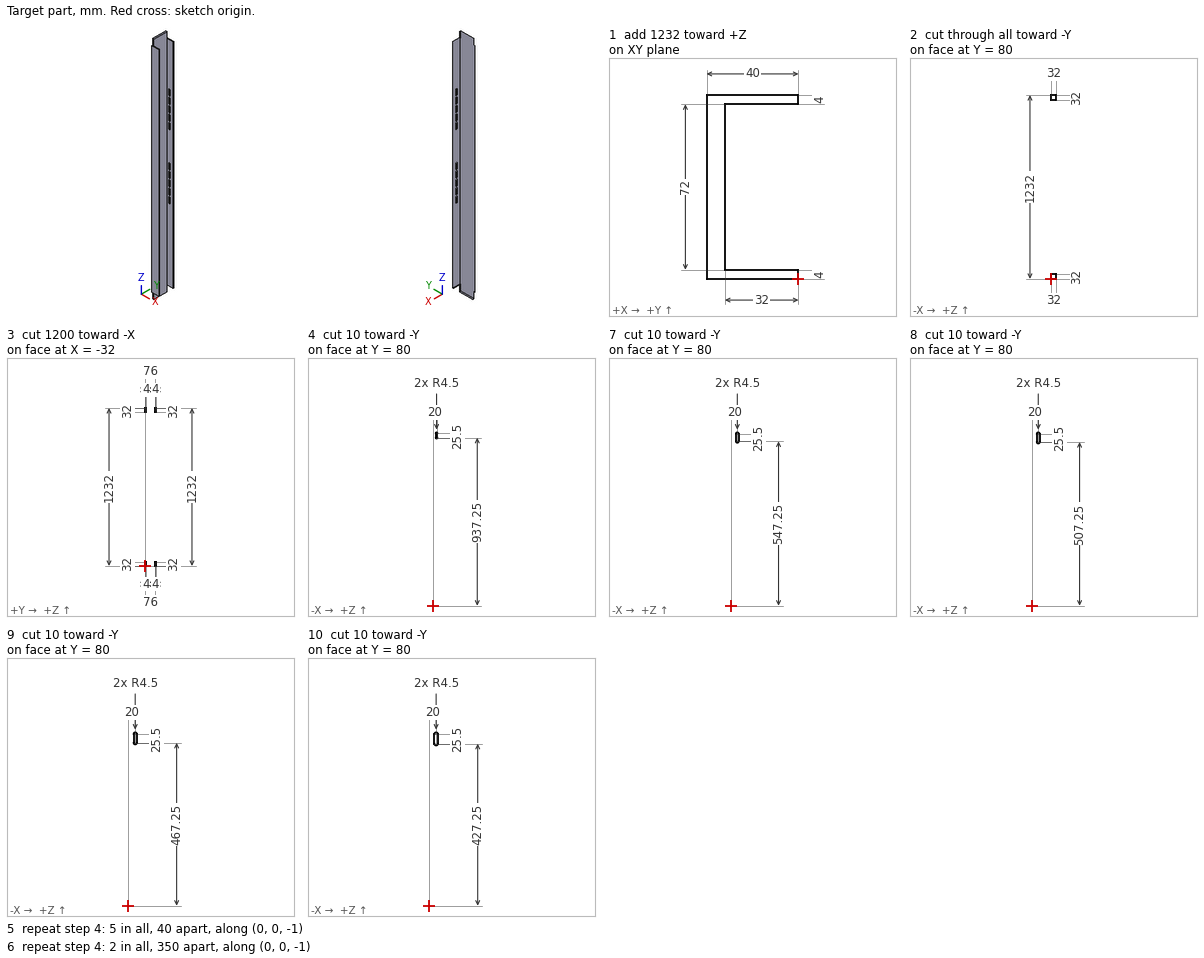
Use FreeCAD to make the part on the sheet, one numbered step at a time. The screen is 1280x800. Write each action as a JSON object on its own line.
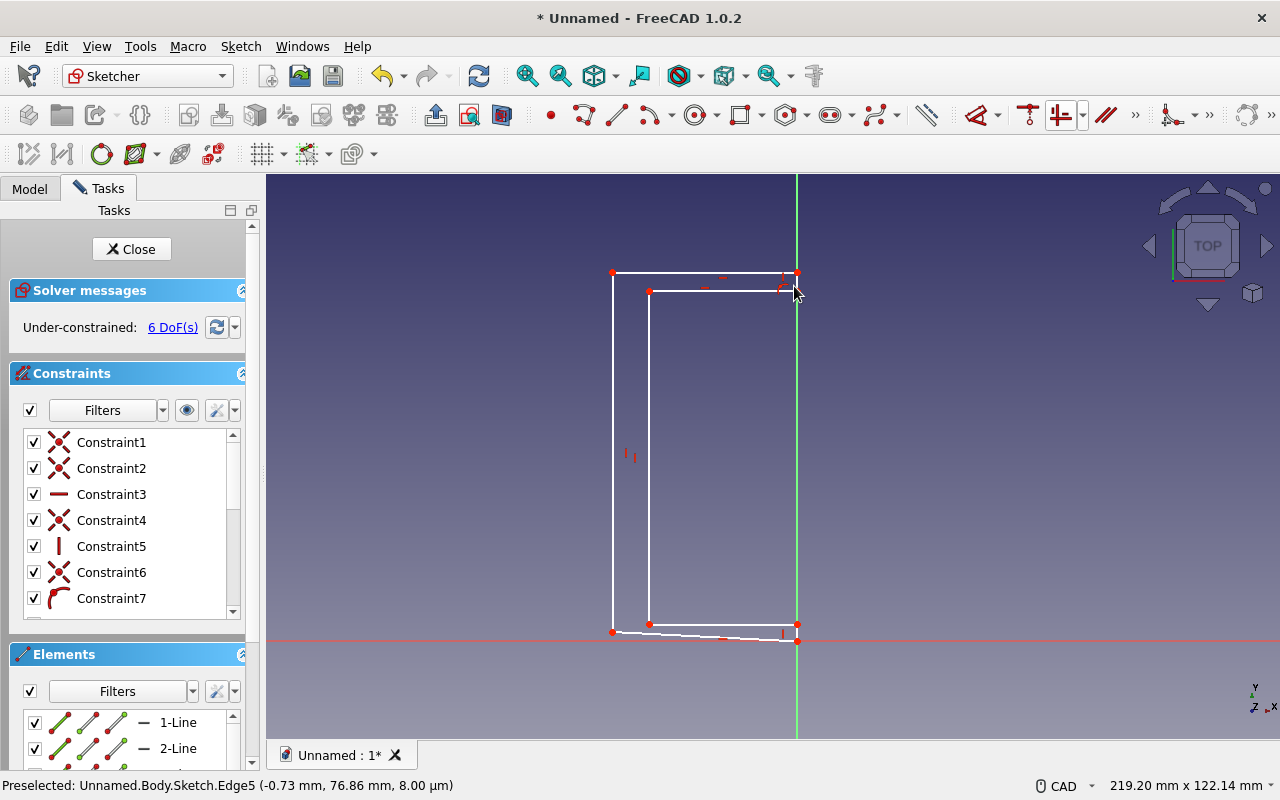
{"action": "scroll", "coordinate": [668, 635], "scroll_direction": "up", "scroll_amount": 4}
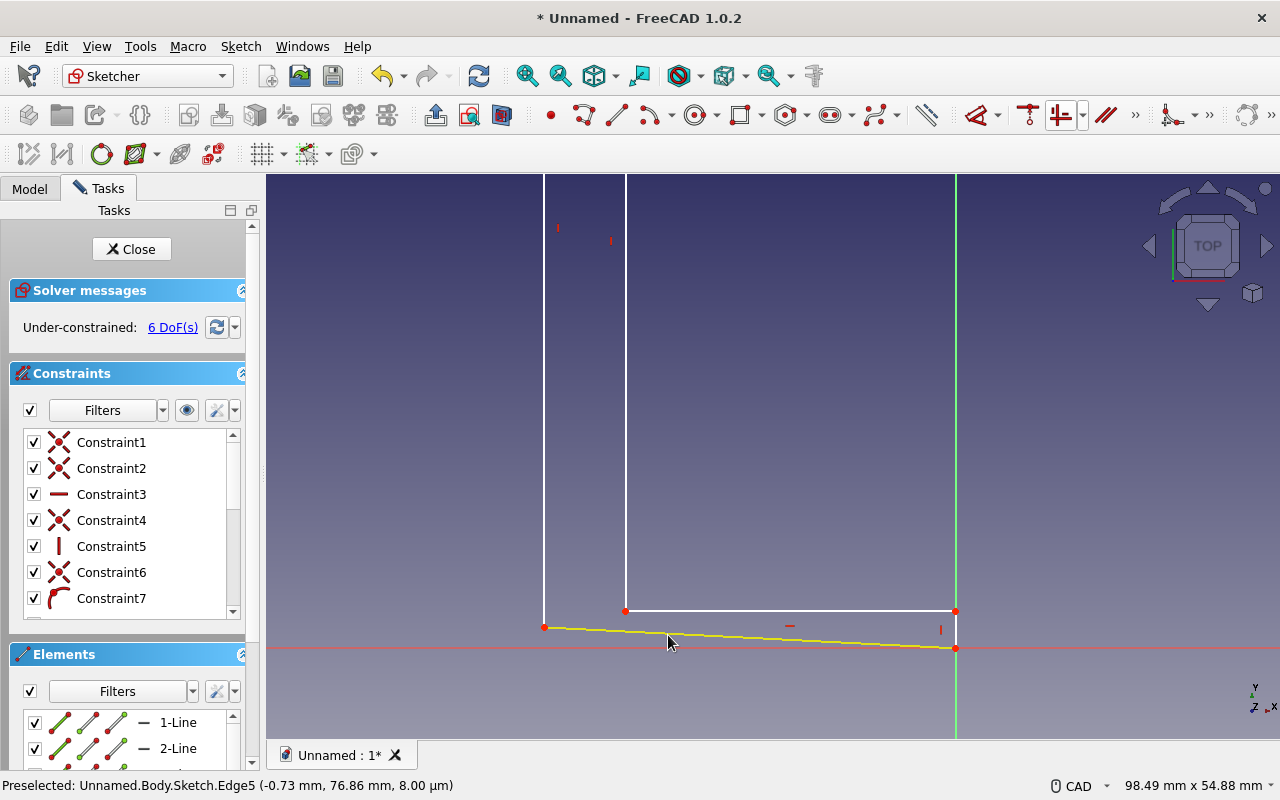
{"action": "left_click", "coordinate": [668, 634]}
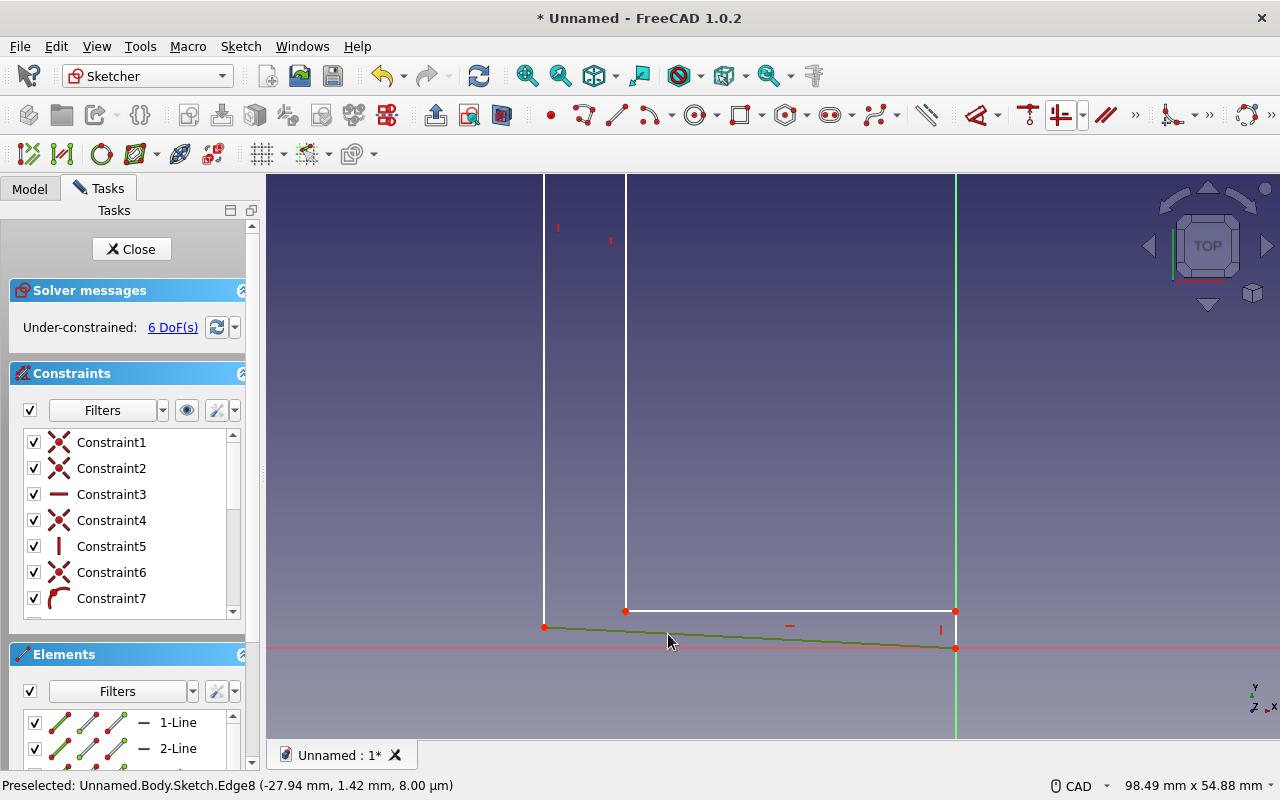
{"action": "left_click", "coordinate": [1082, 116]}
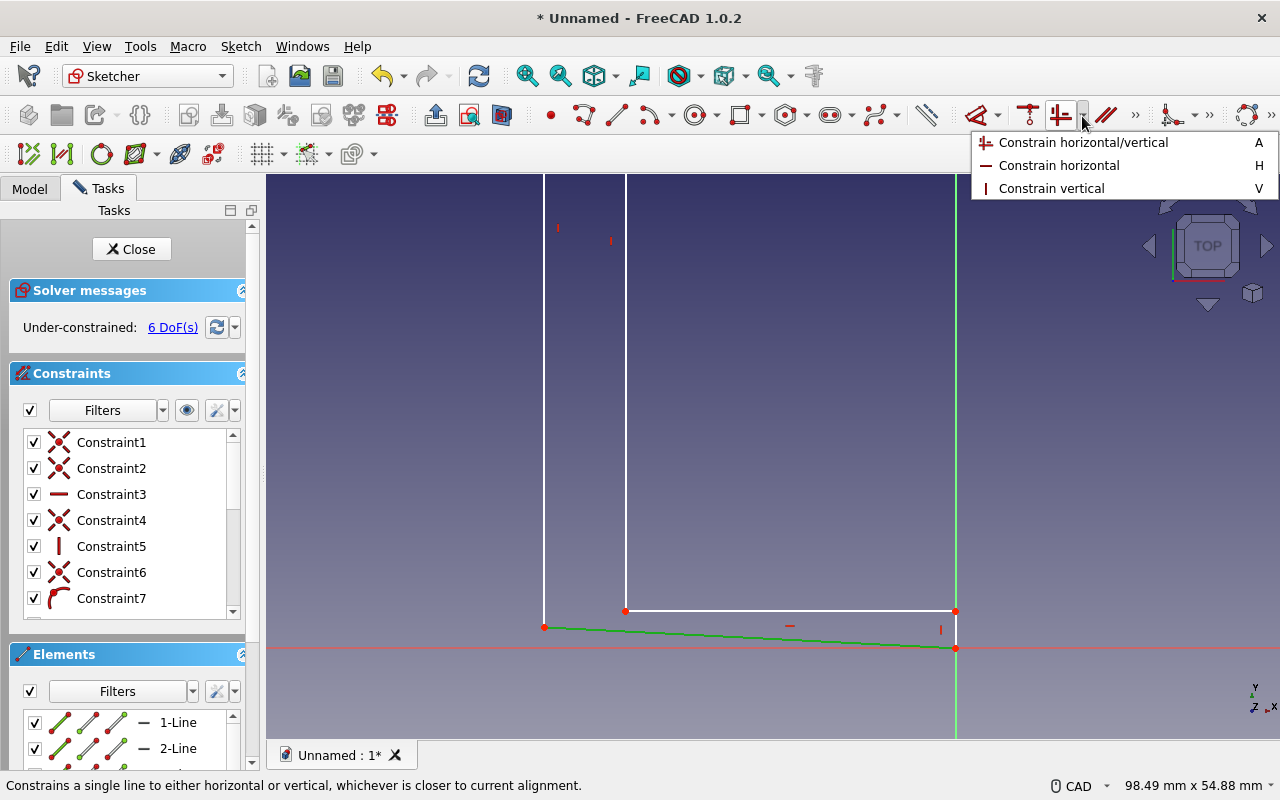
{"action": "left_click", "coordinate": [1125, 166]}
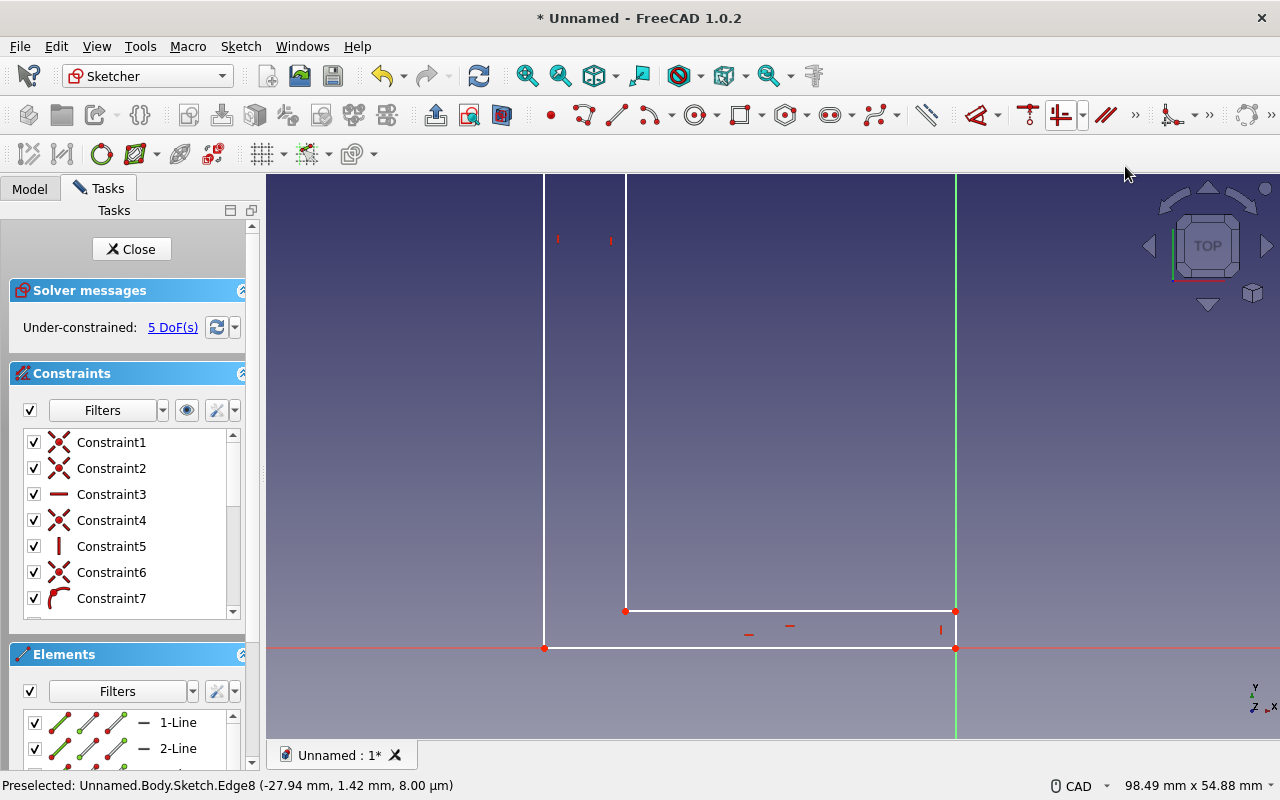
{"action": "scroll", "coordinate": [956, 637], "scroll_direction": "up", "scroll_amount": 2}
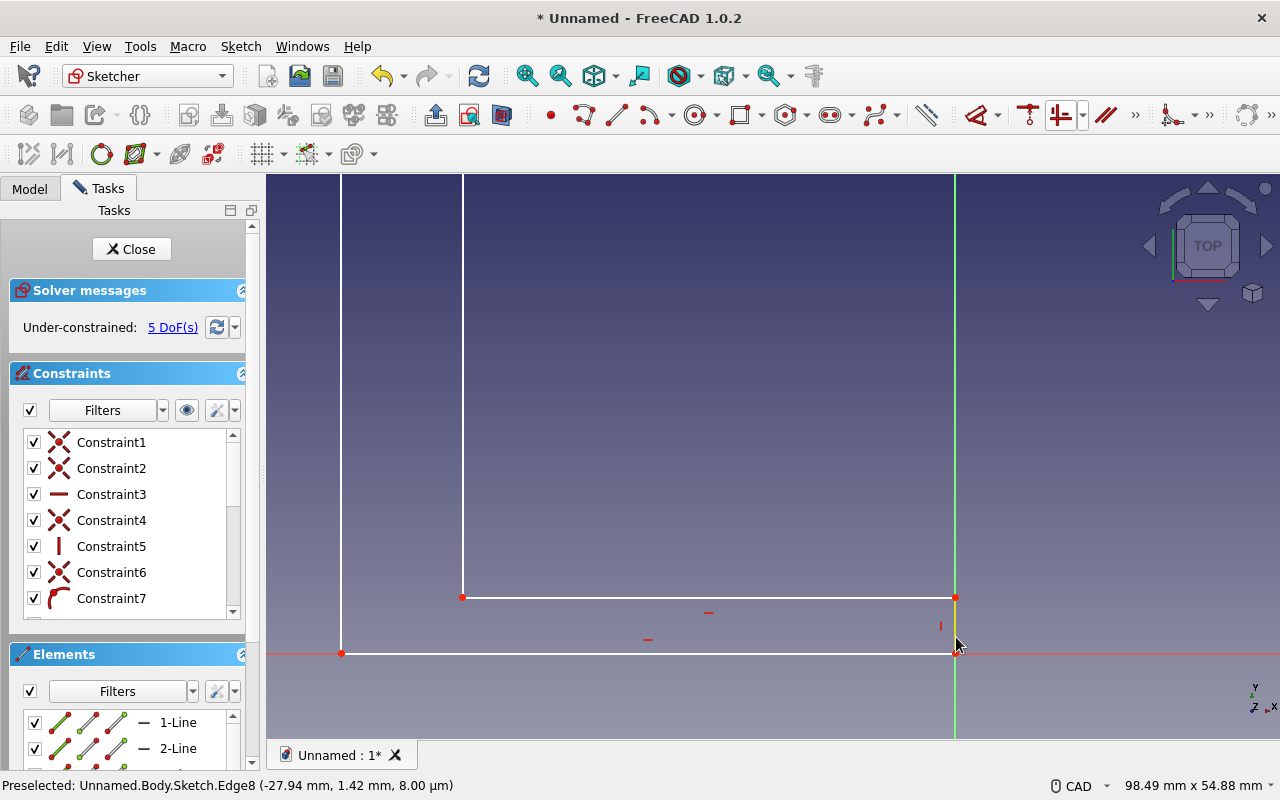
{"action": "left_click", "coordinate": [955, 637]}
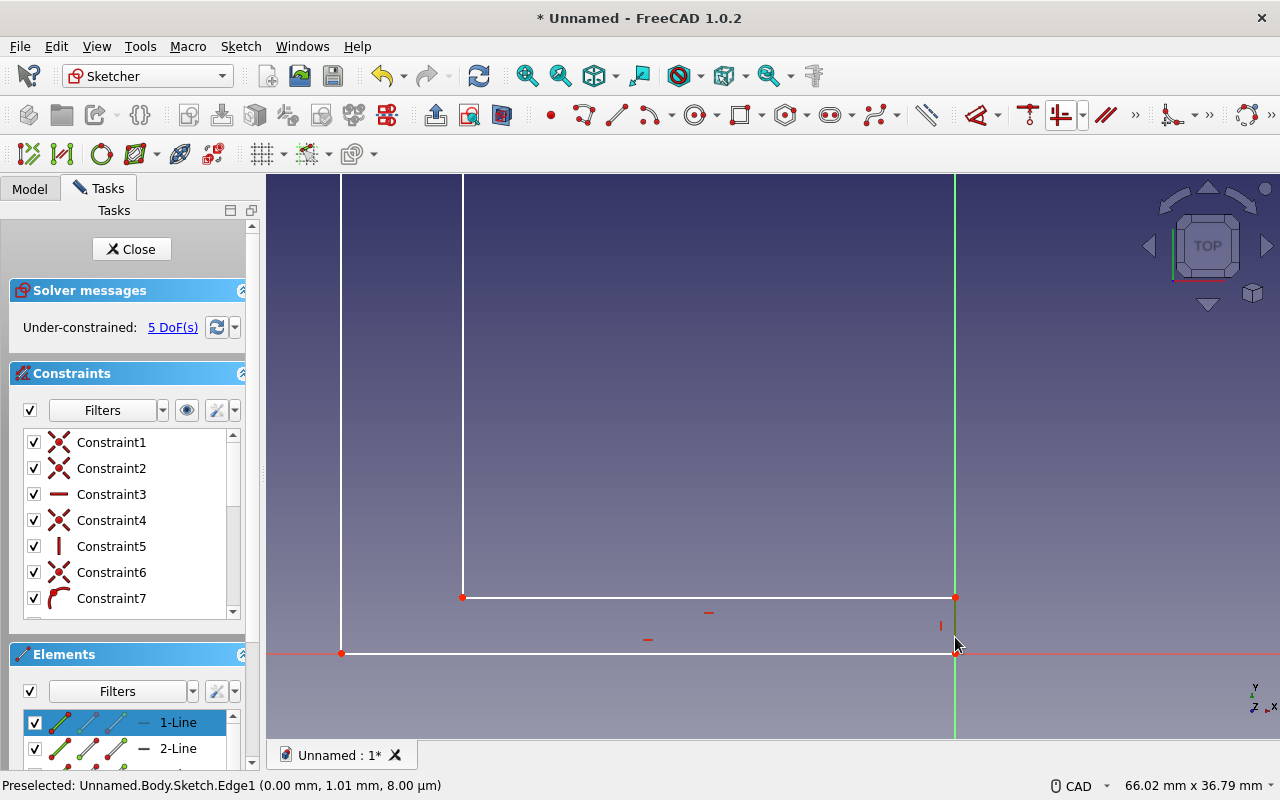
{"action": "left_click", "coordinate": [998, 116]}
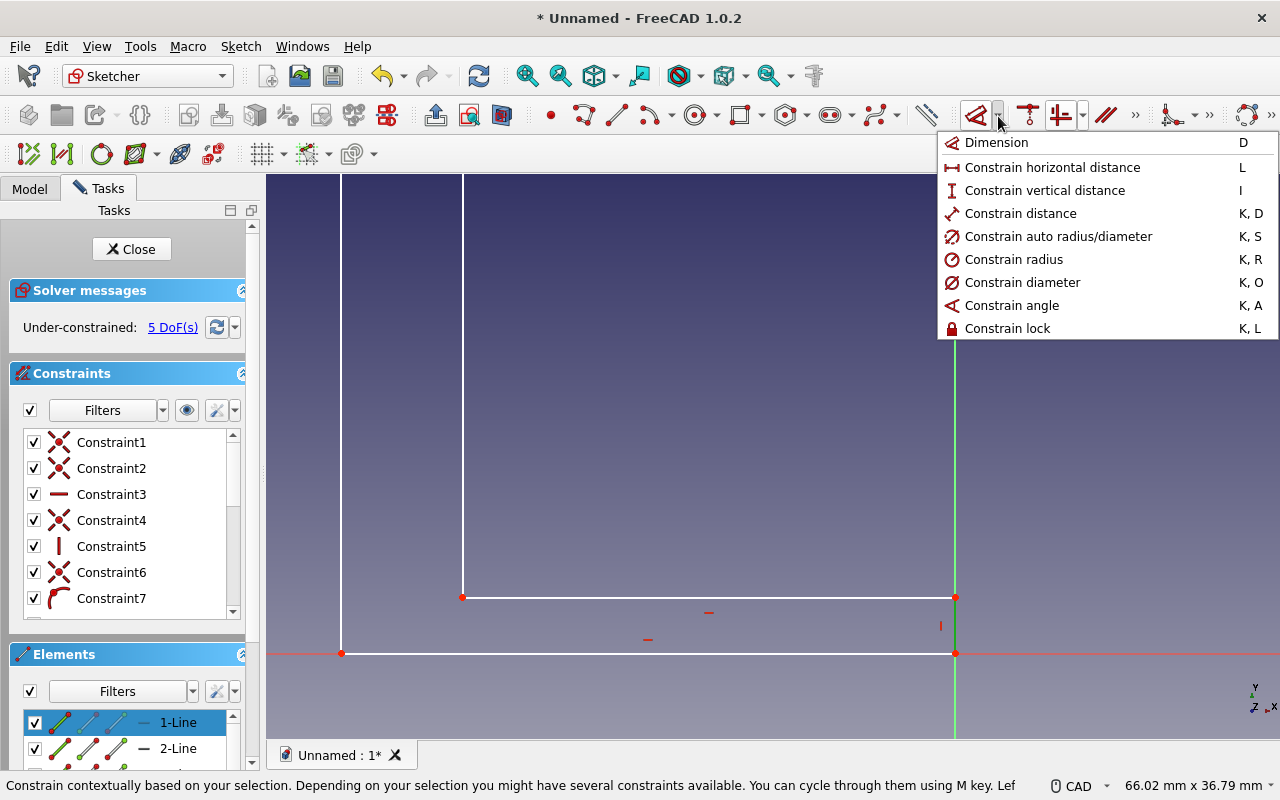
{"action": "left_click", "coordinate": [1108, 190]}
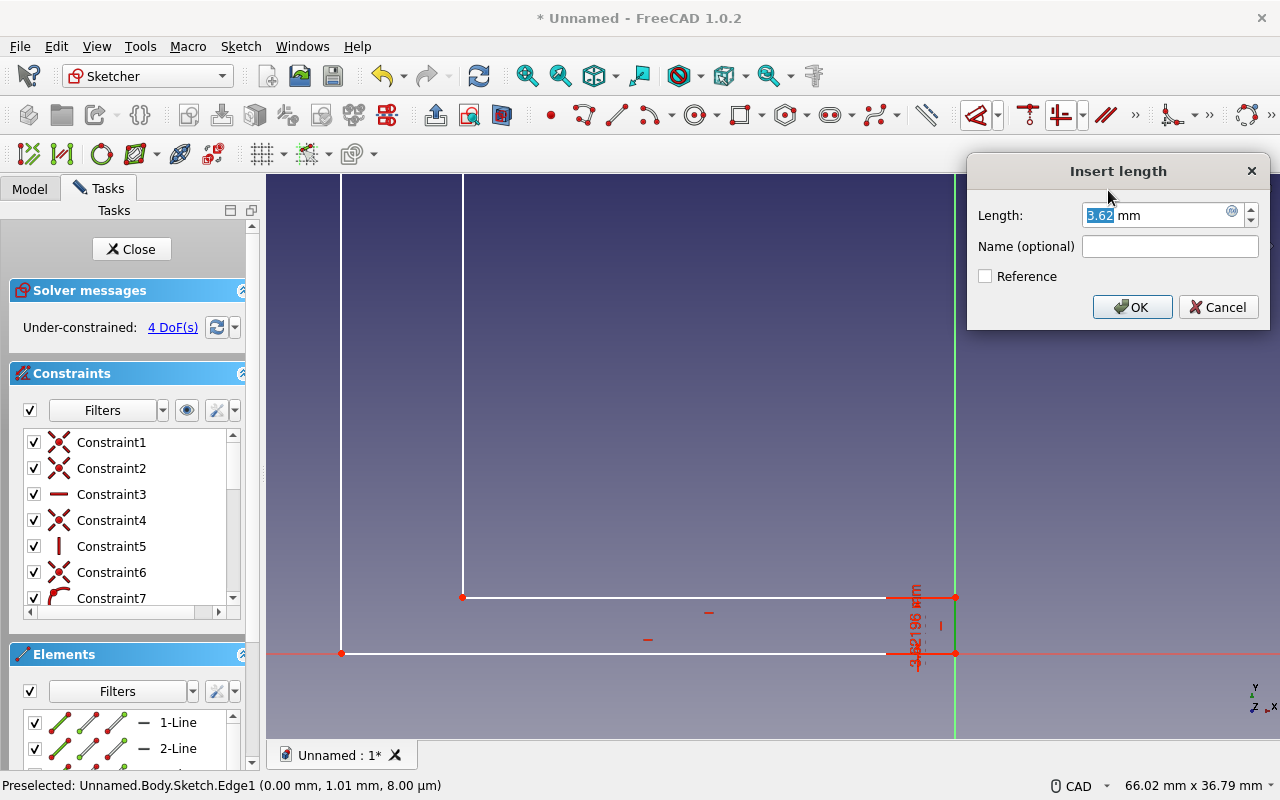
{"action": "type", "text": "4"}
{"action": "key", "text": "Return"}